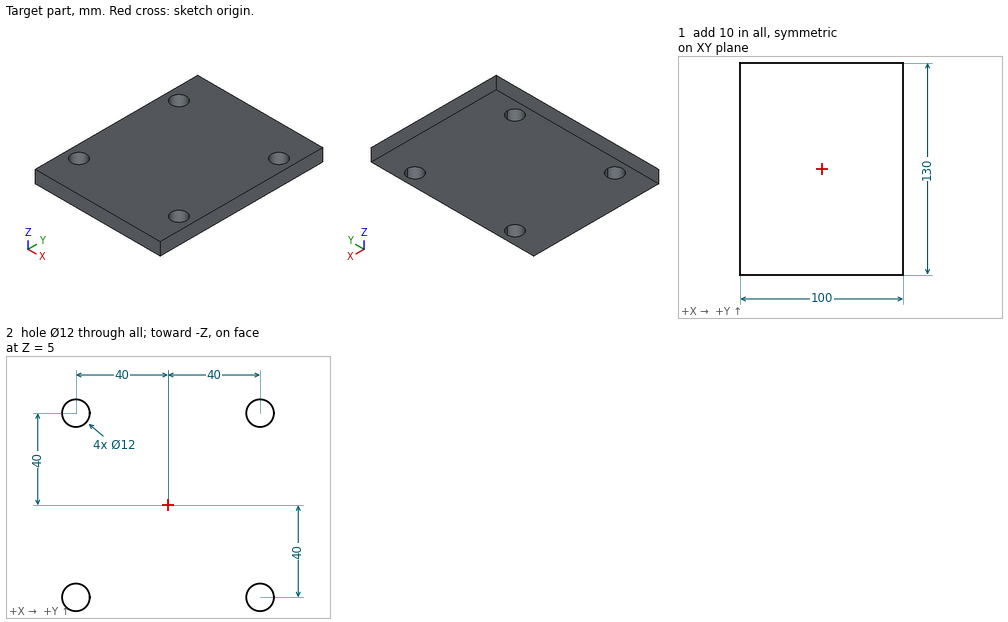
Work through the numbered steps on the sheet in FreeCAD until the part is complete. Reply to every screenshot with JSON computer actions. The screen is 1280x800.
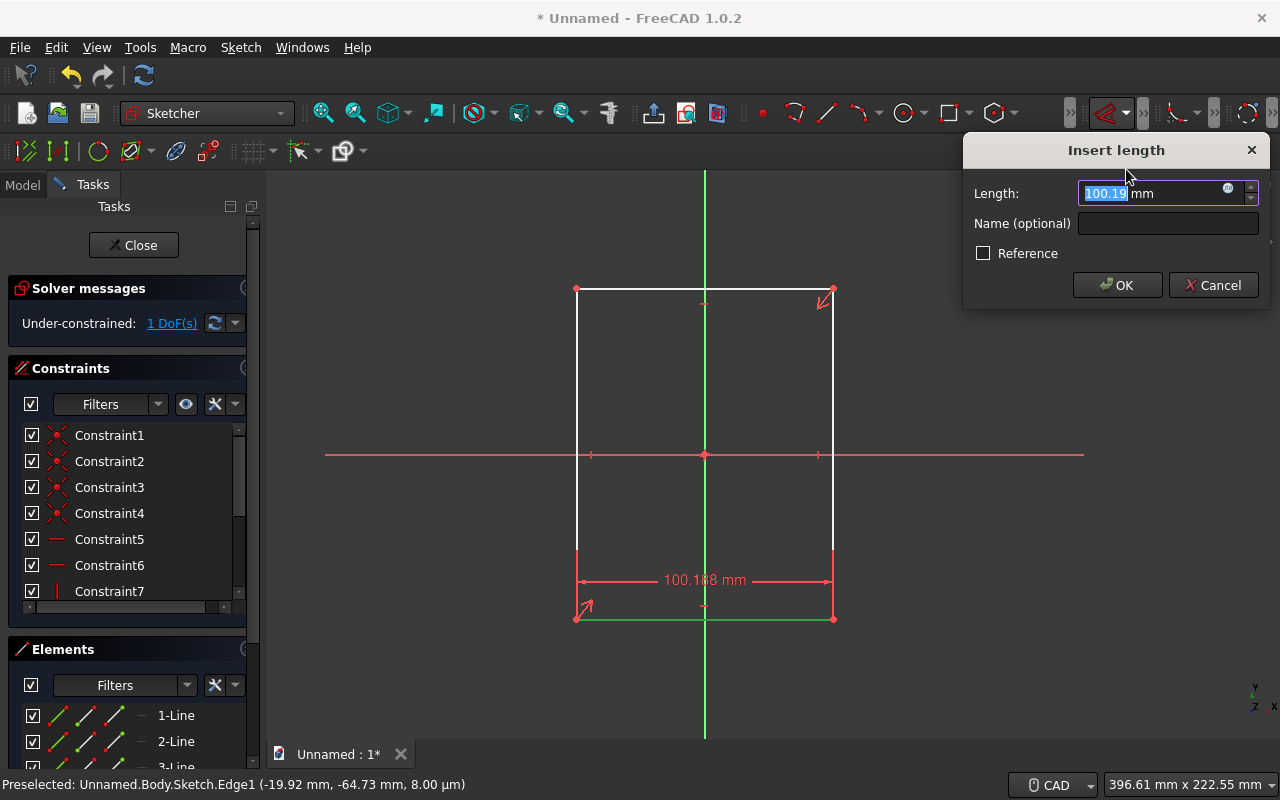
{"action": "type", "text": "100"}
{"action": "key", "text": "Return"}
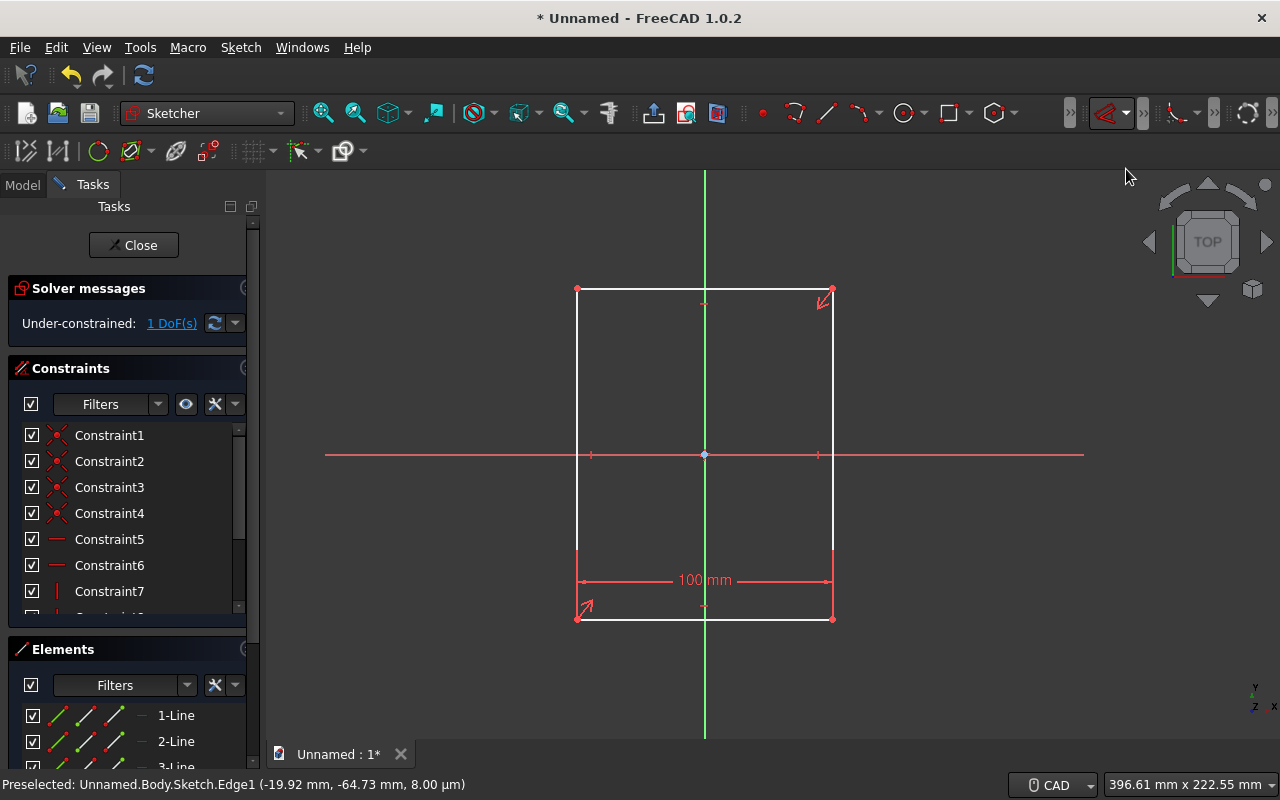
{"action": "left_click", "coordinate": [833, 521]}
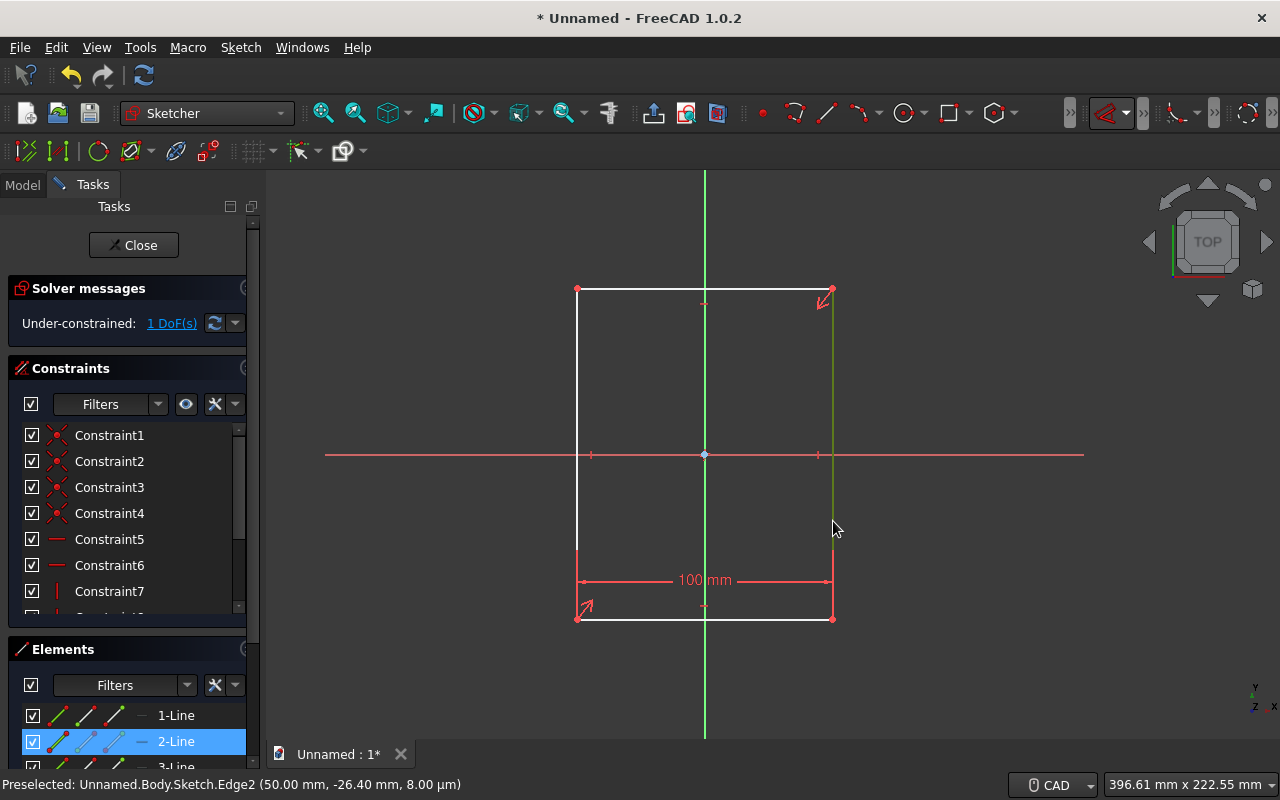
{"action": "key", "text": "i"}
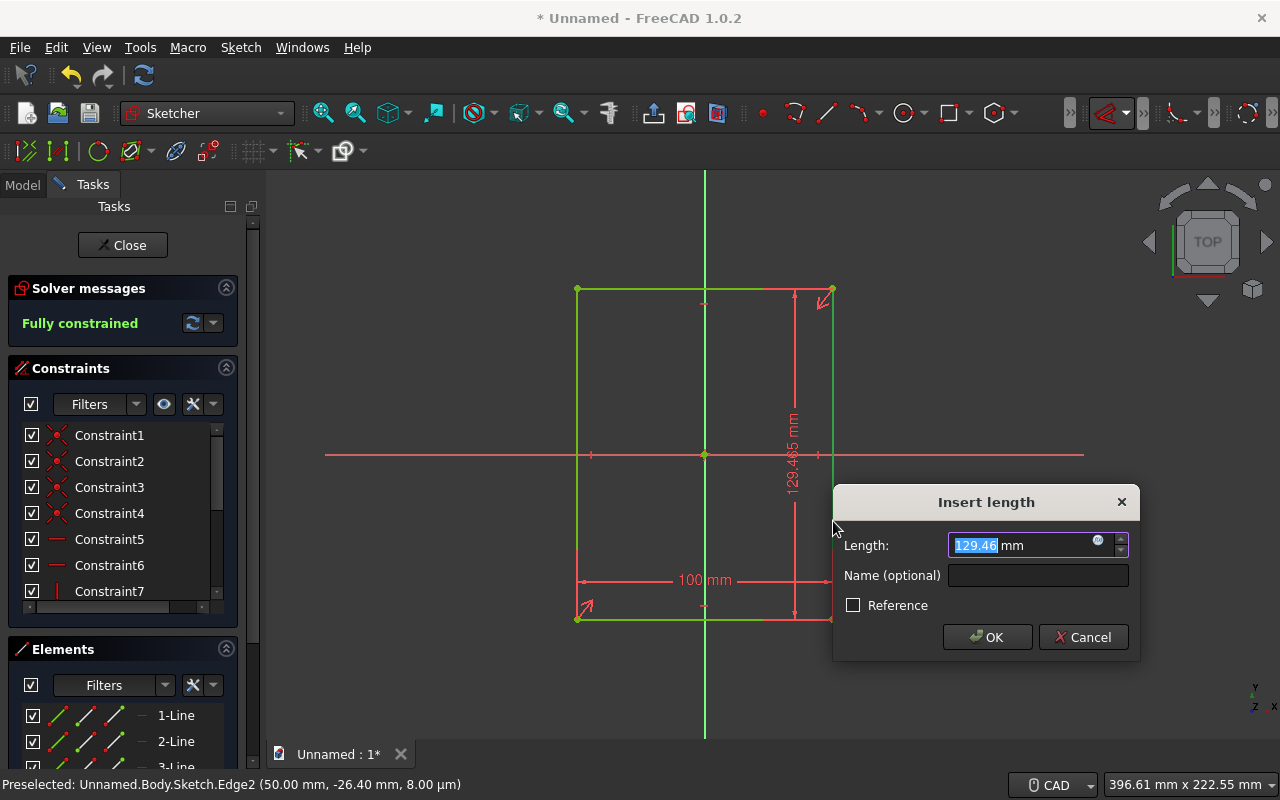
{"action": "type", "text": "130"}
{"action": "key", "text": "Return"}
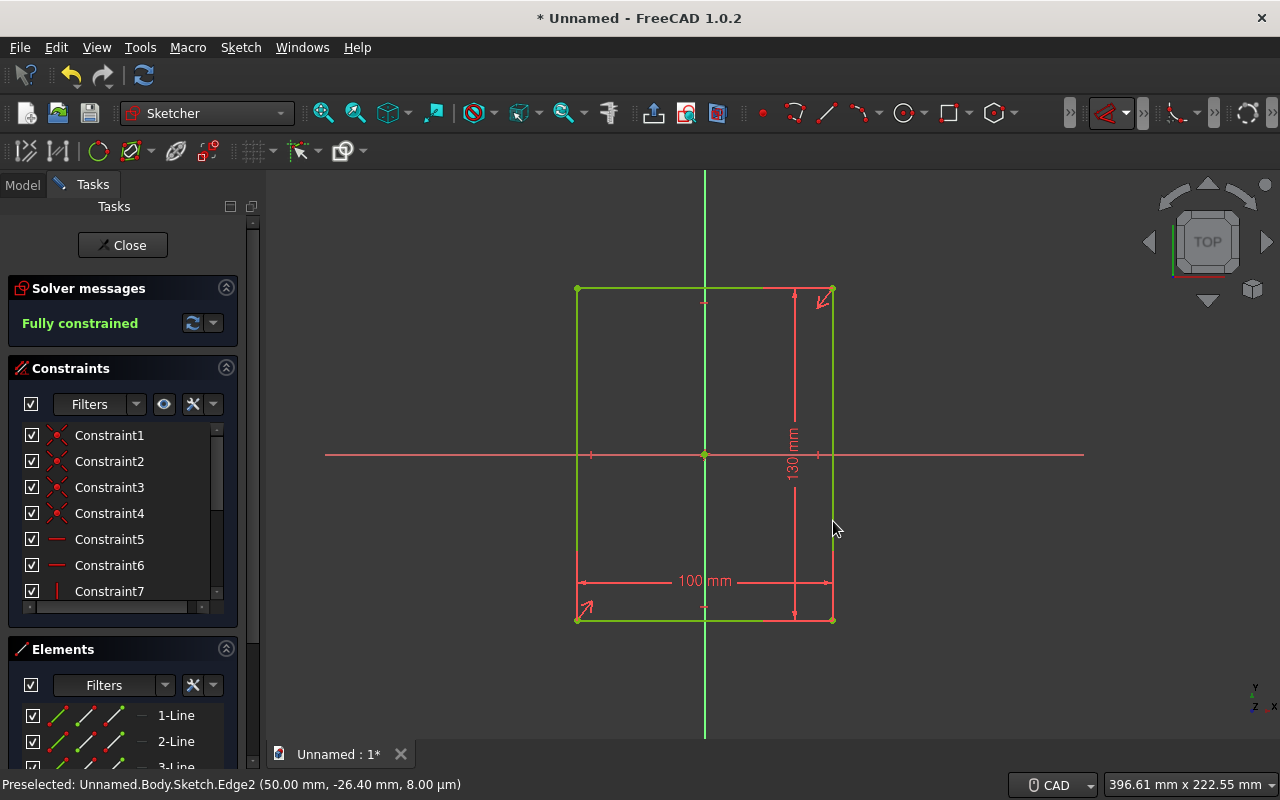
{"action": "left_click", "coordinate": [123, 245]}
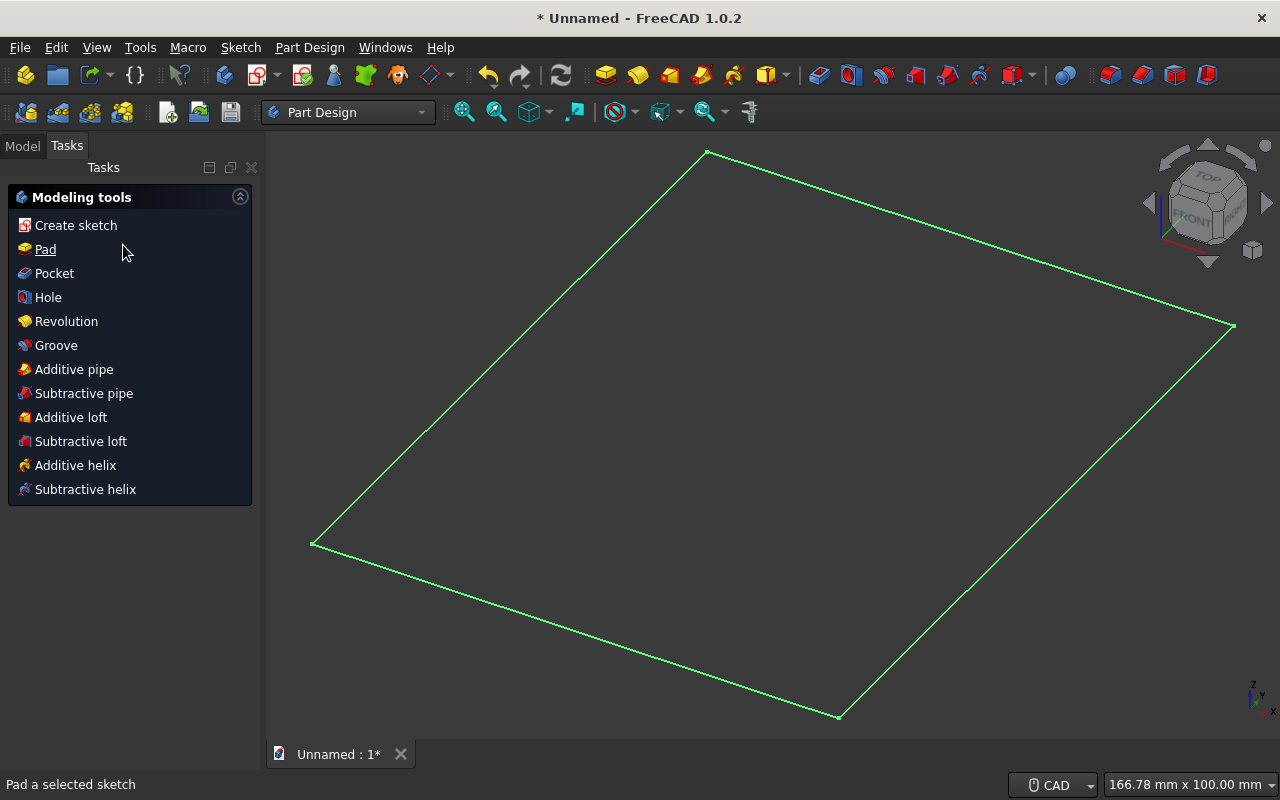
{"action": "left_click", "coordinate": [606, 76]}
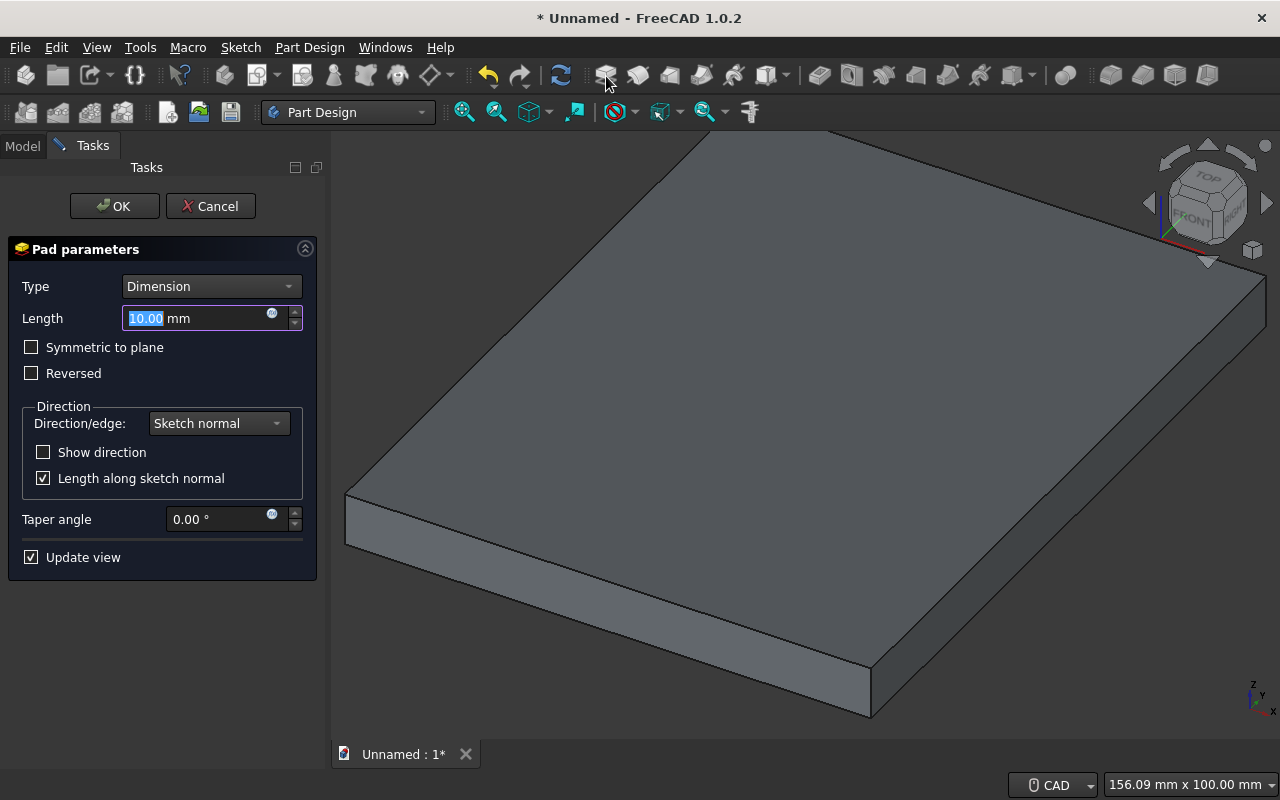
{"action": "type", "text": "10"}
{"action": "key", "text": "Tab"}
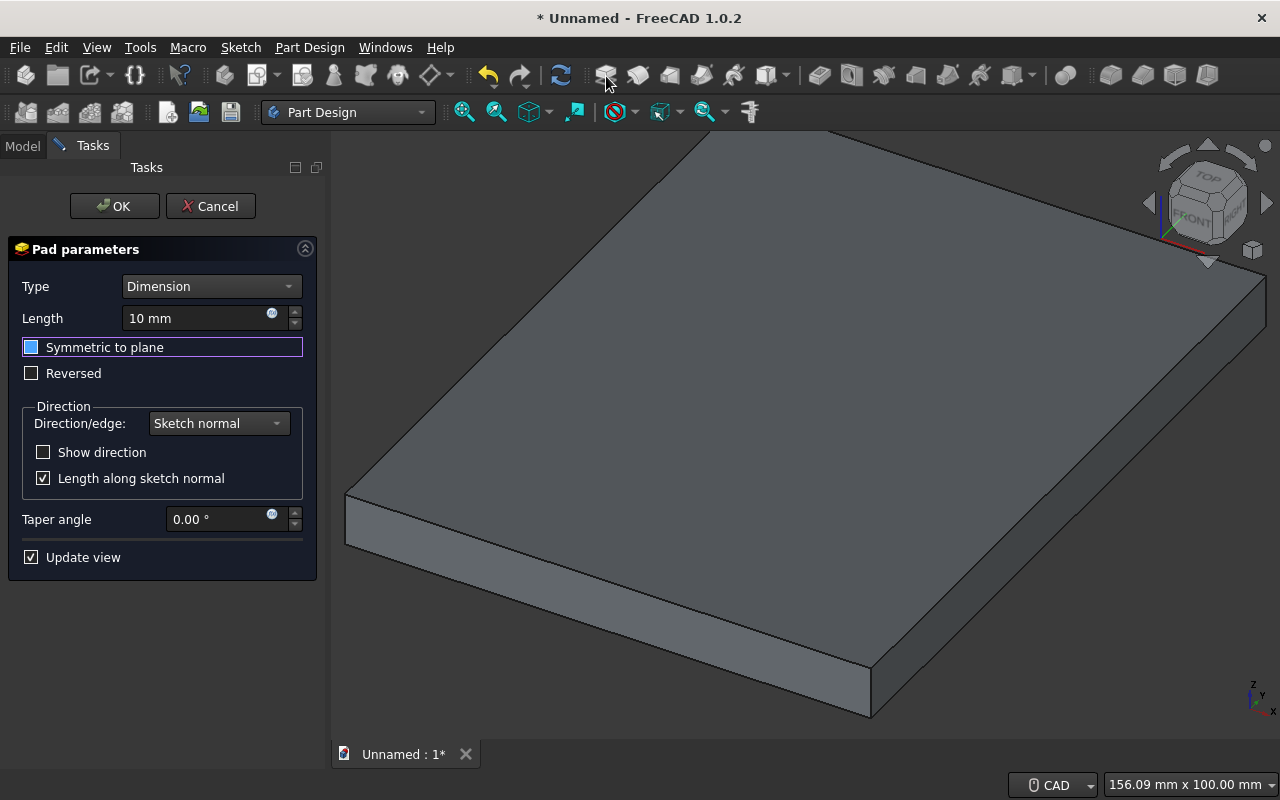
{"action": "left_click", "coordinate": [30, 347]}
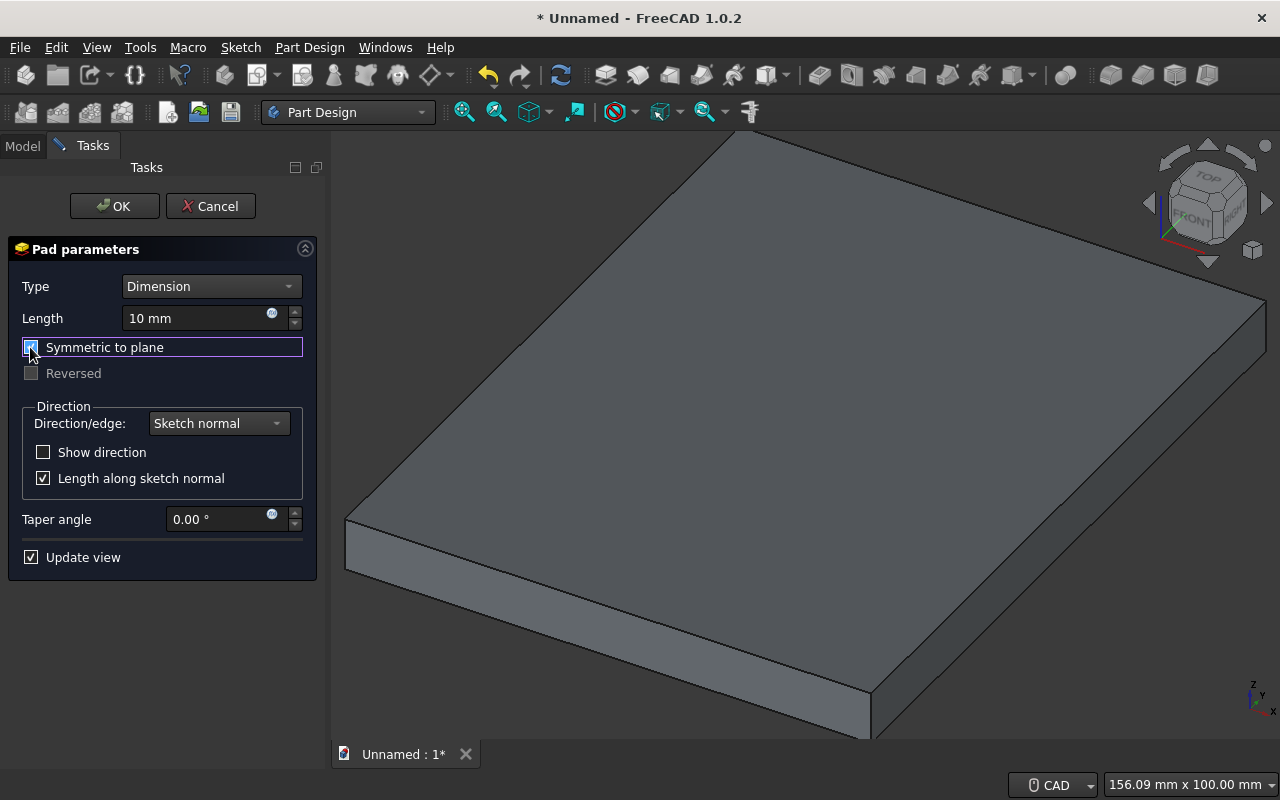
{"action": "left_click", "coordinate": [115, 206]}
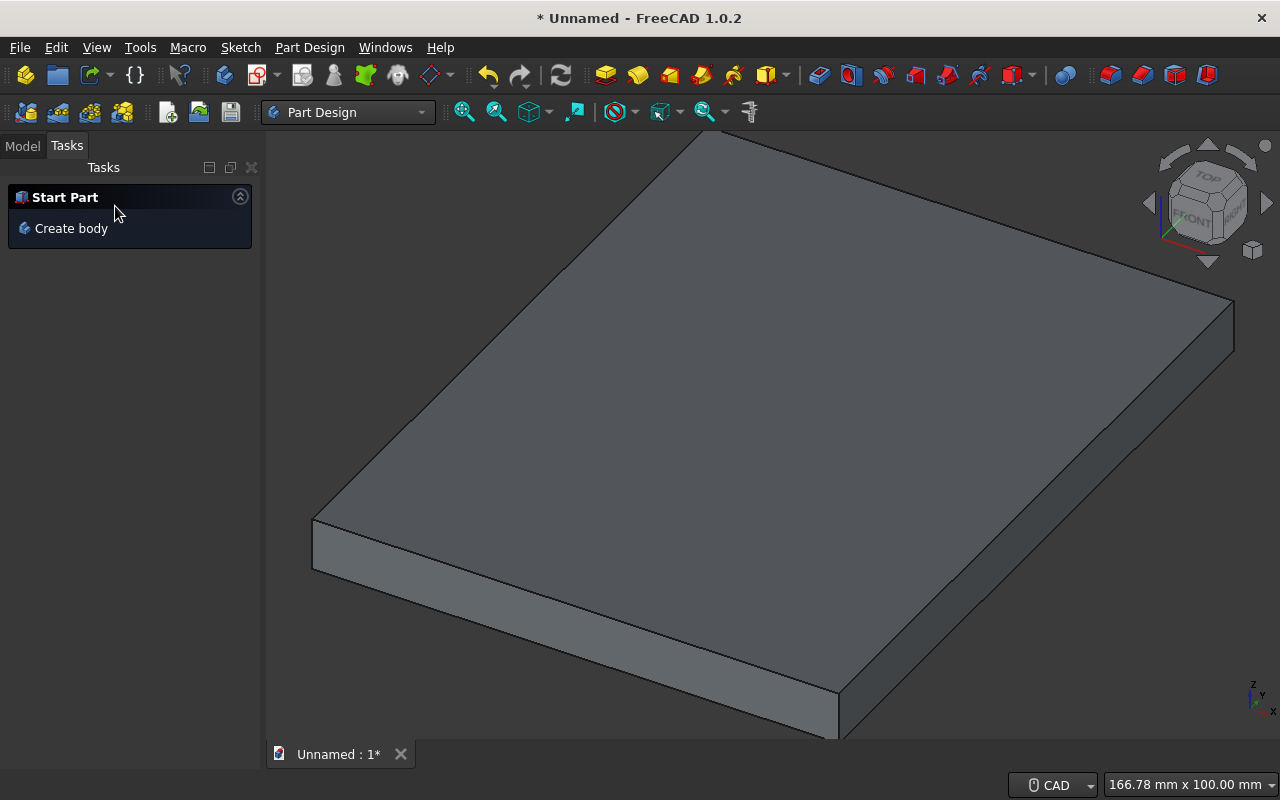
{"action": "key", "text": "v f"}